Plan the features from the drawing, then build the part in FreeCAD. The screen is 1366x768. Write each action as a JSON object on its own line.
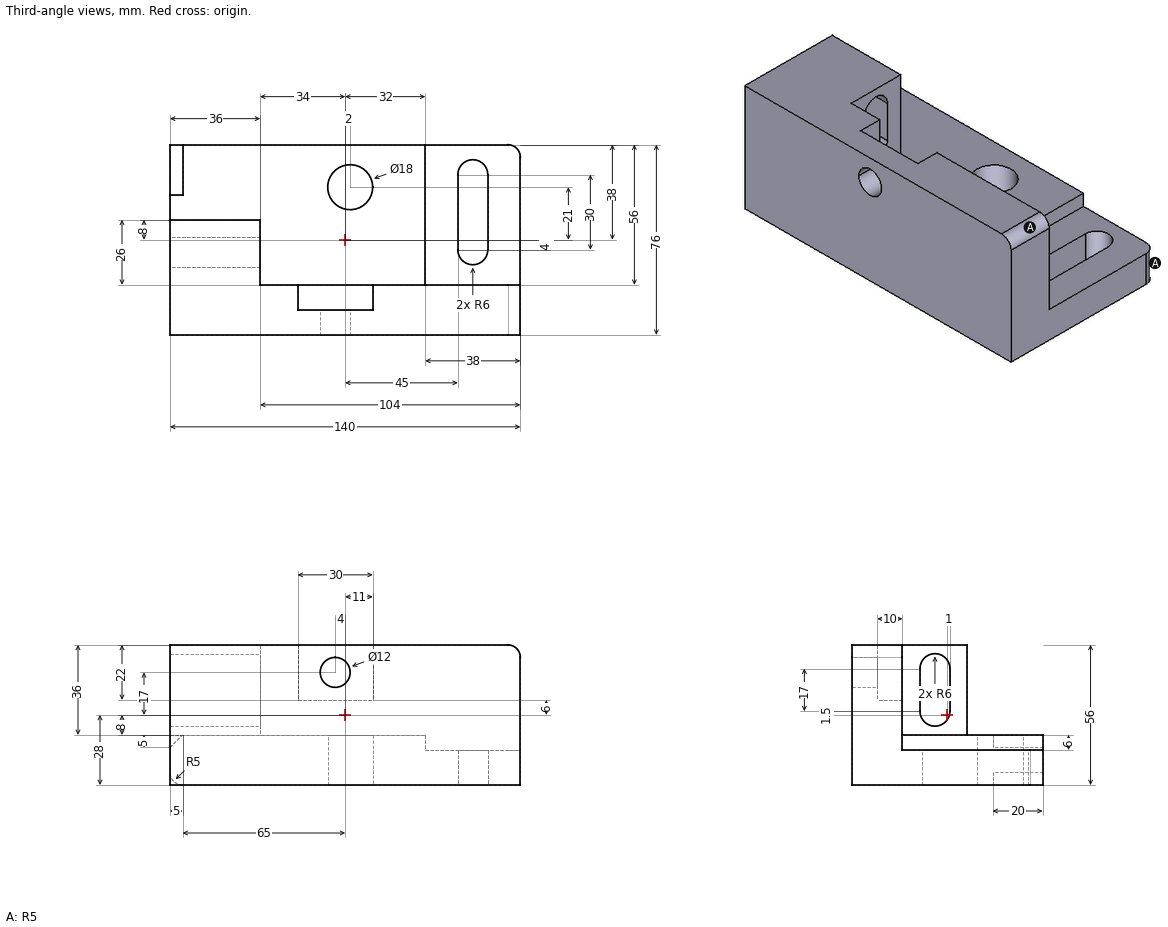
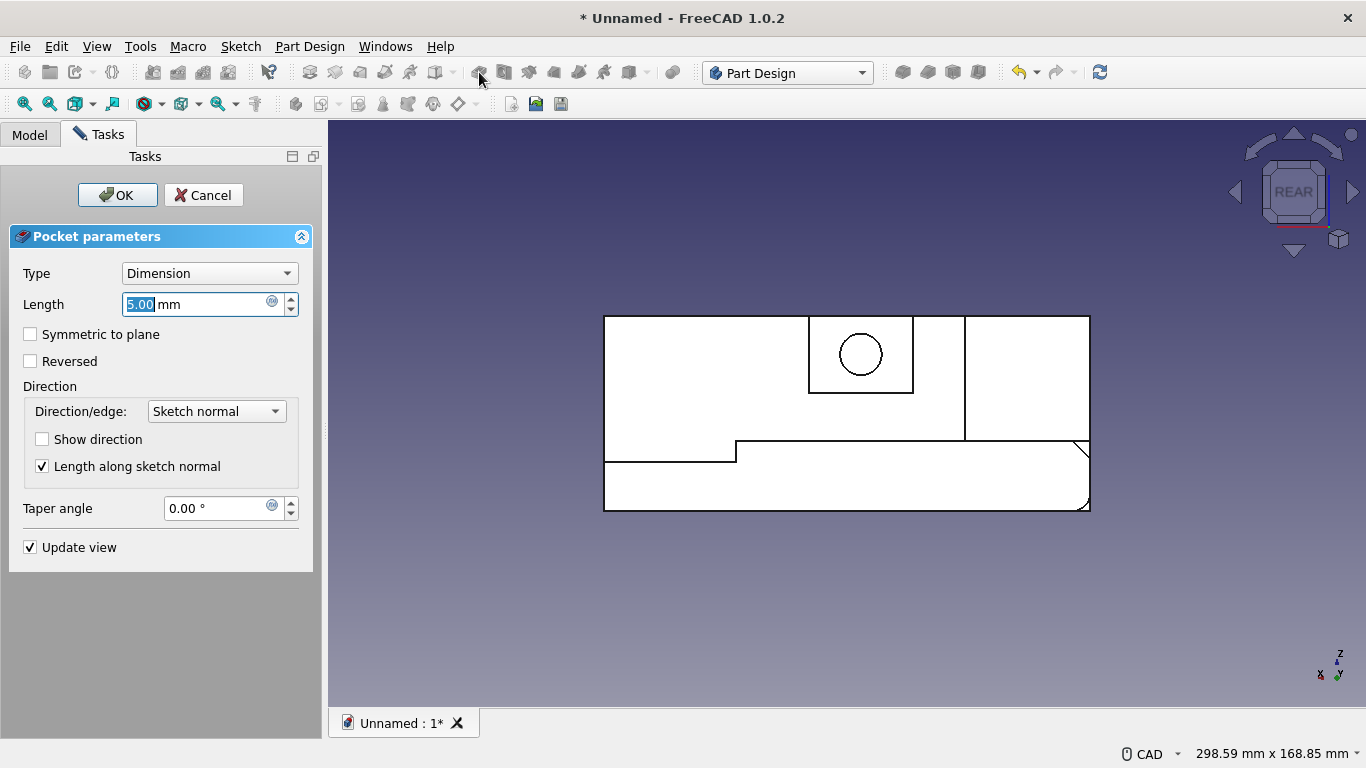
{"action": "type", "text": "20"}
{"action": "key", "text": "Tab"}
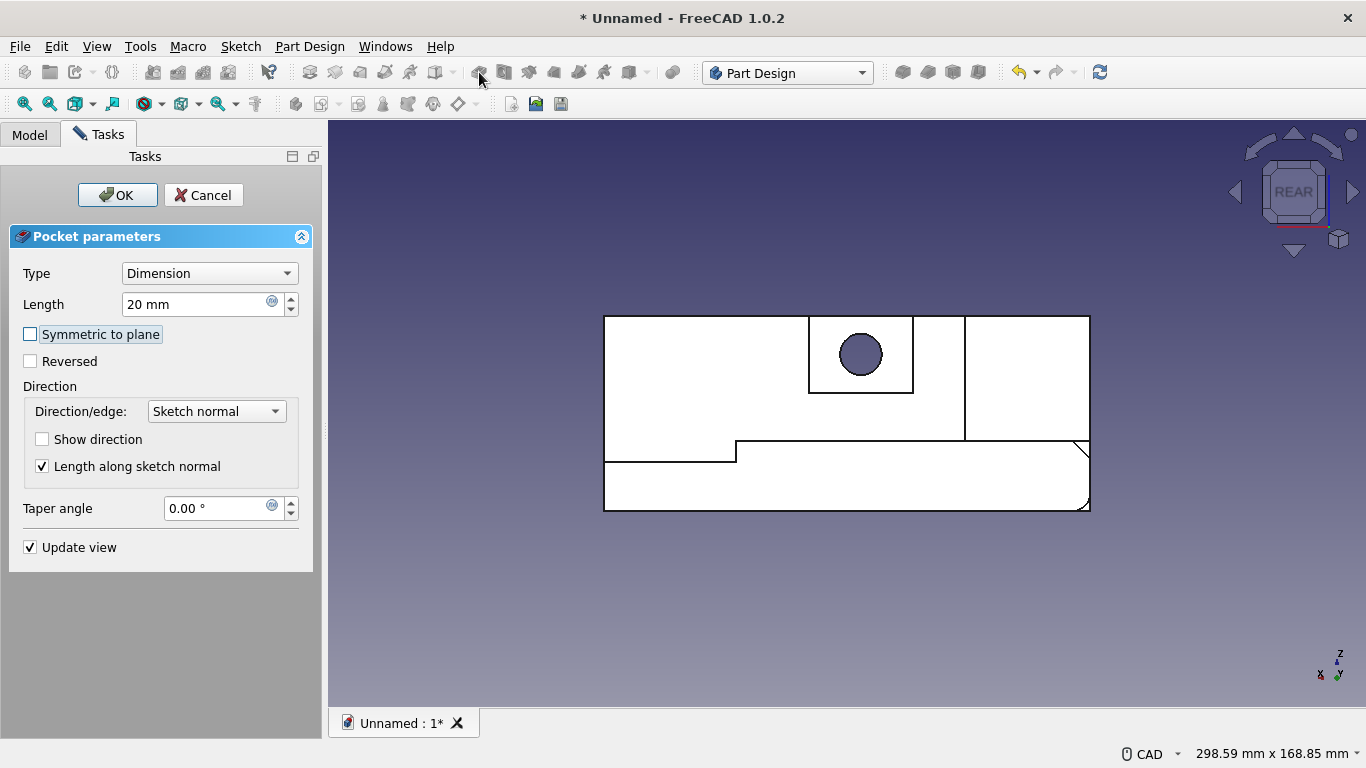
{"action": "left_click", "coordinate": [118, 195]}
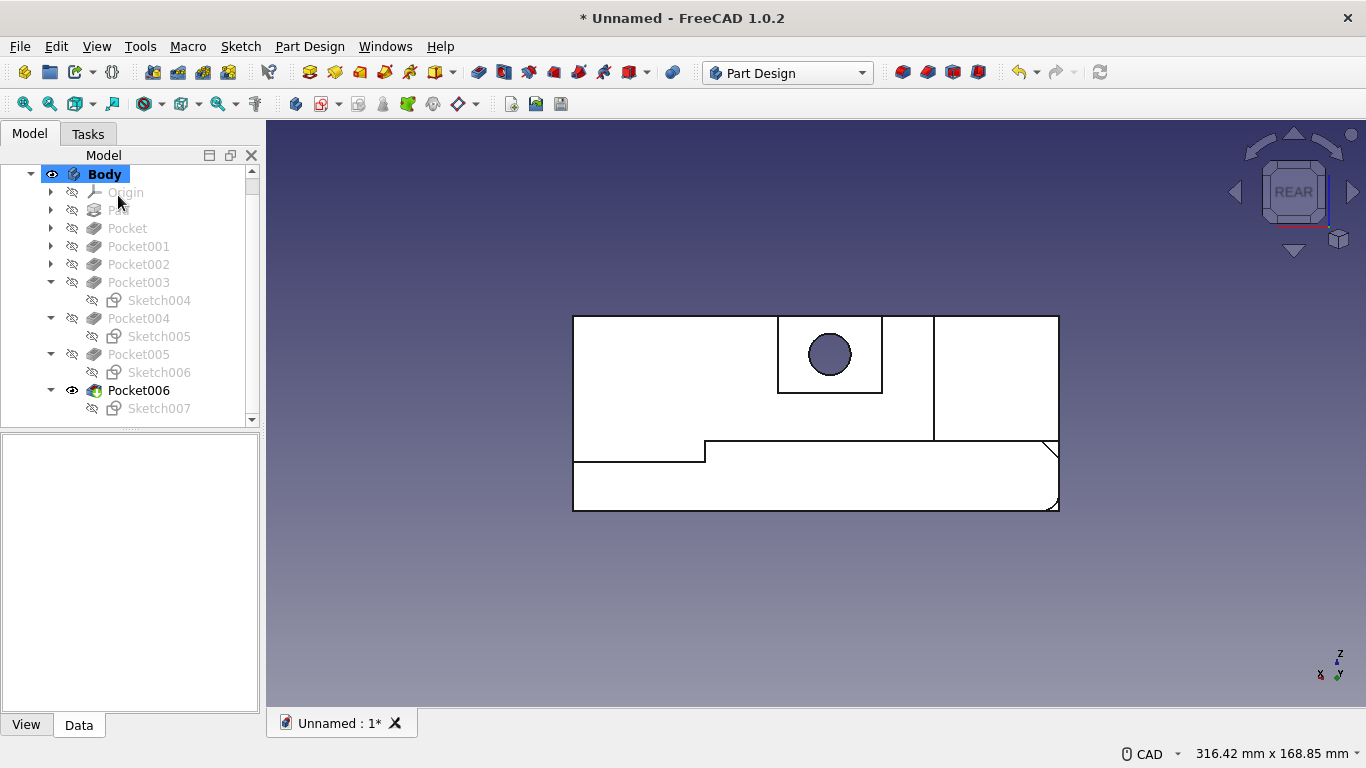
{"action": "left_click", "coordinate": [25, 104]}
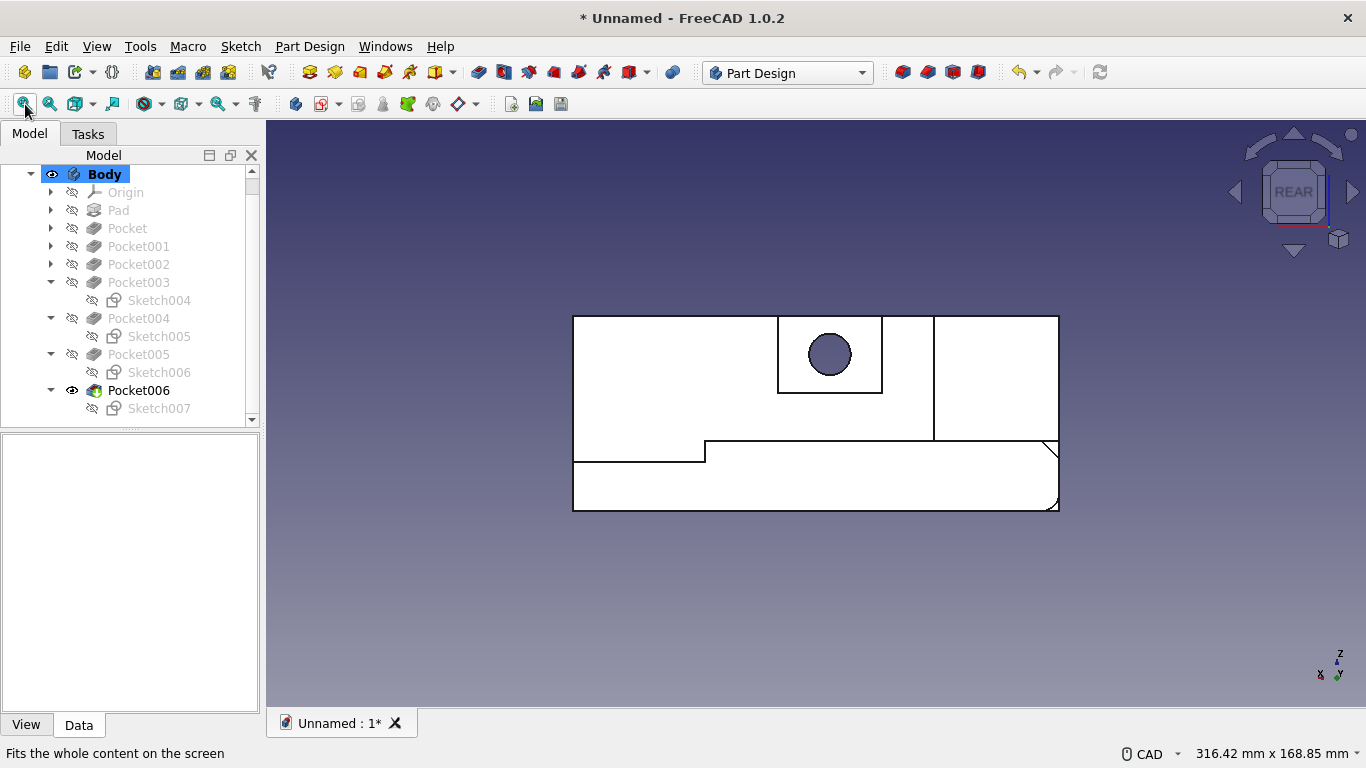
{"action": "key", "text": "0"}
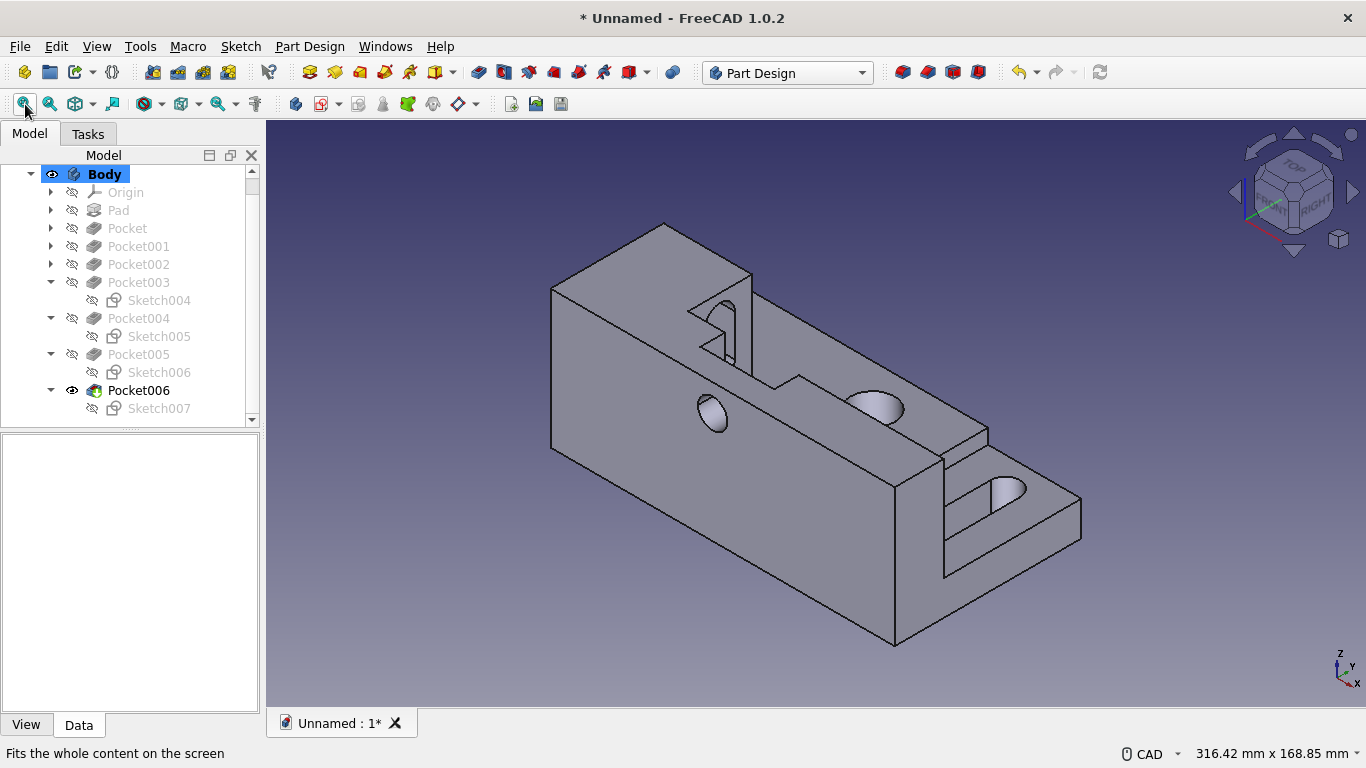
{"action": "left_click", "coordinate": [919, 472]}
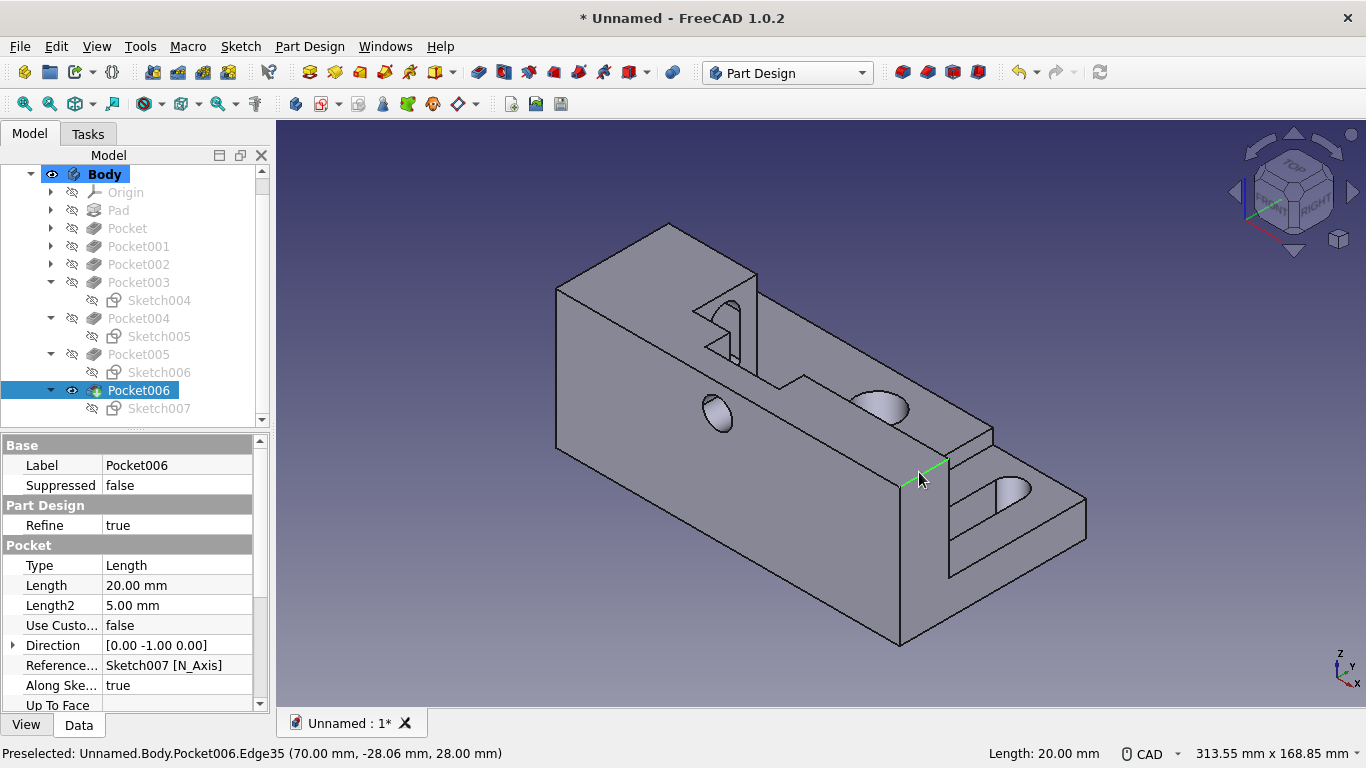
{"action": "key", "text": "2"}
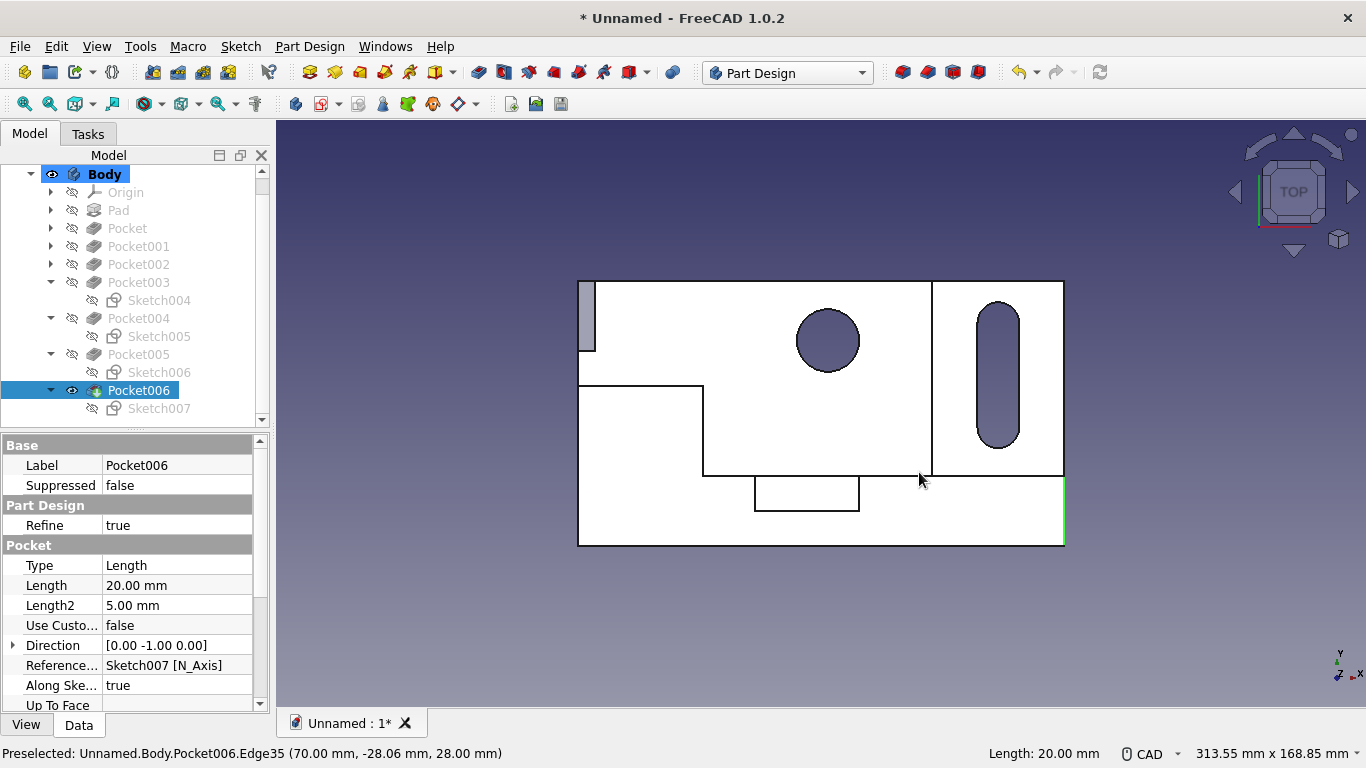
{"action": "key", "text": "1"}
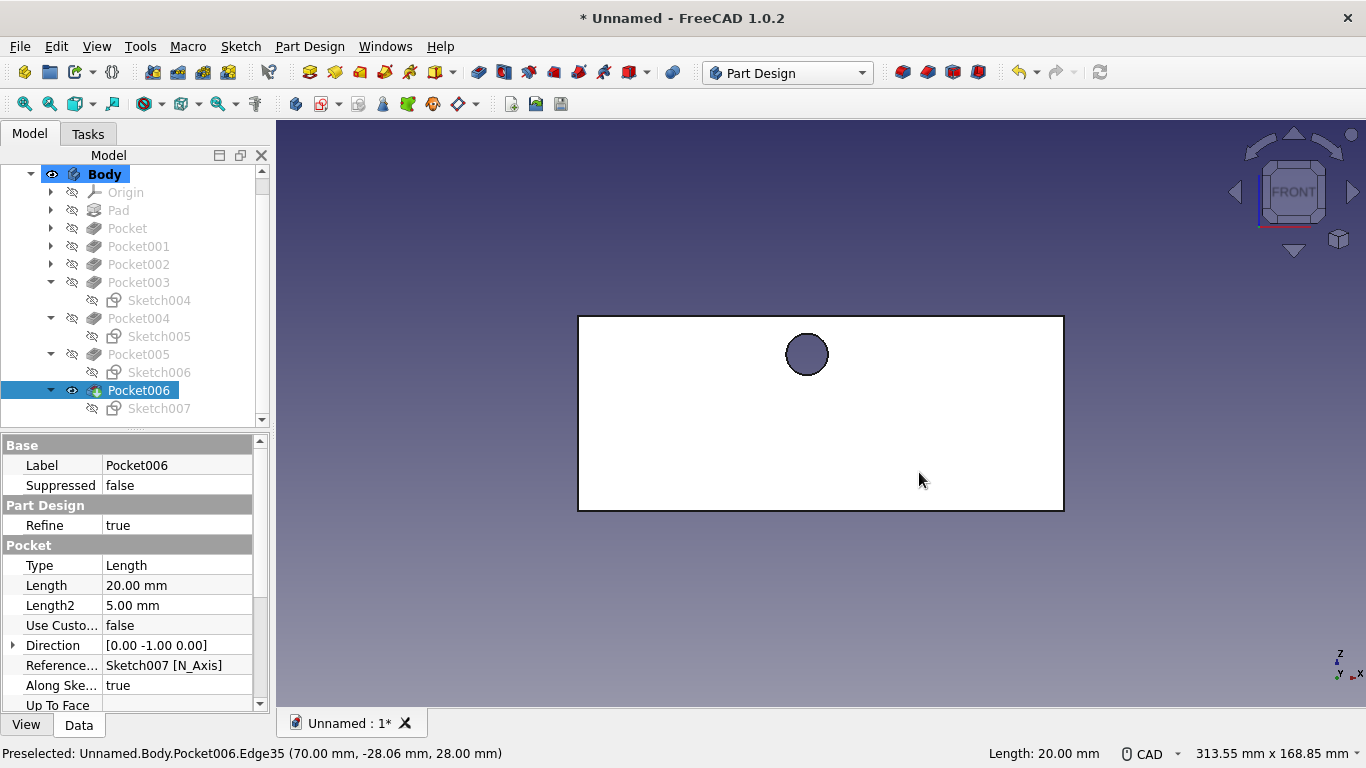
{"action": "key", "text": "v f"}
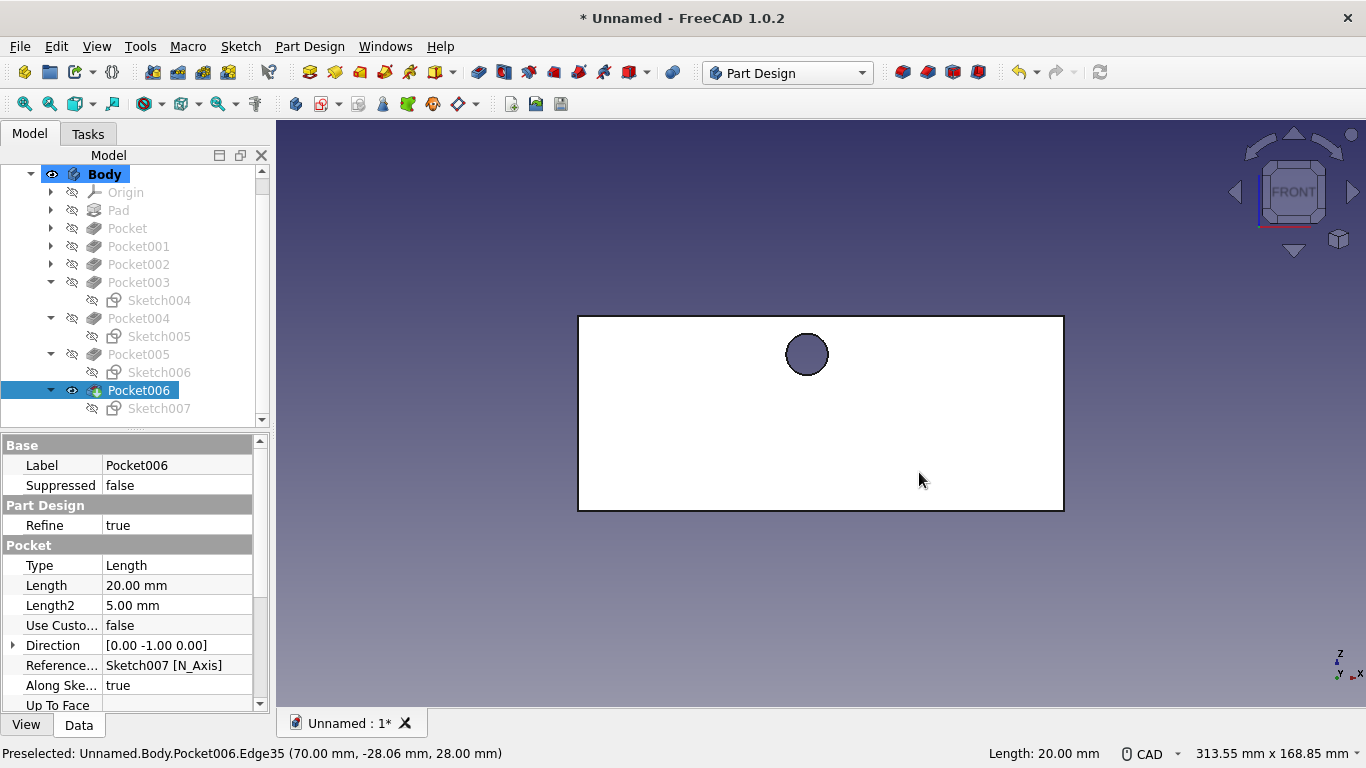
{"action": "key", "text": "3"}